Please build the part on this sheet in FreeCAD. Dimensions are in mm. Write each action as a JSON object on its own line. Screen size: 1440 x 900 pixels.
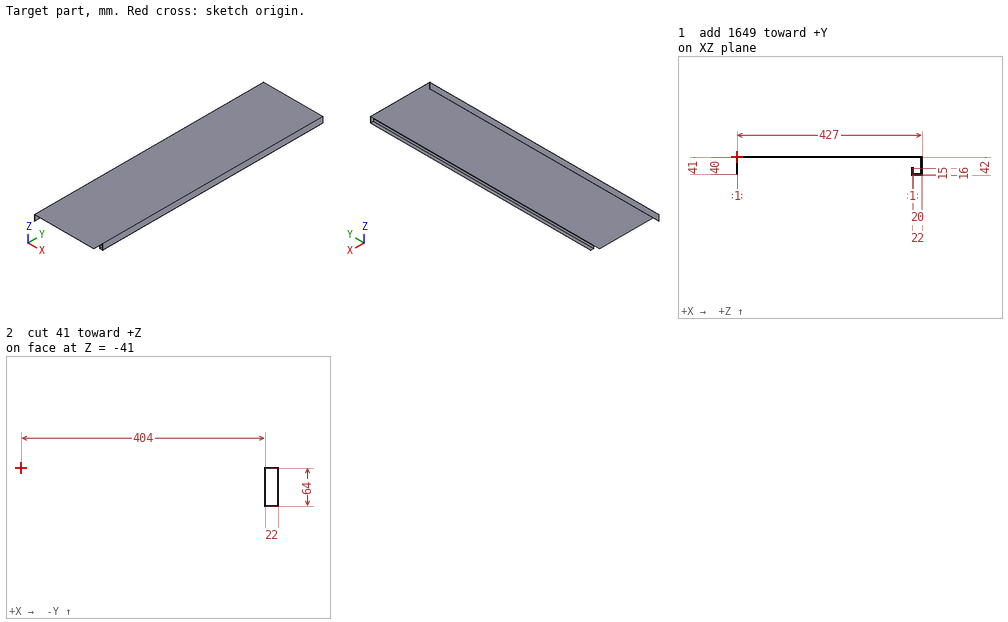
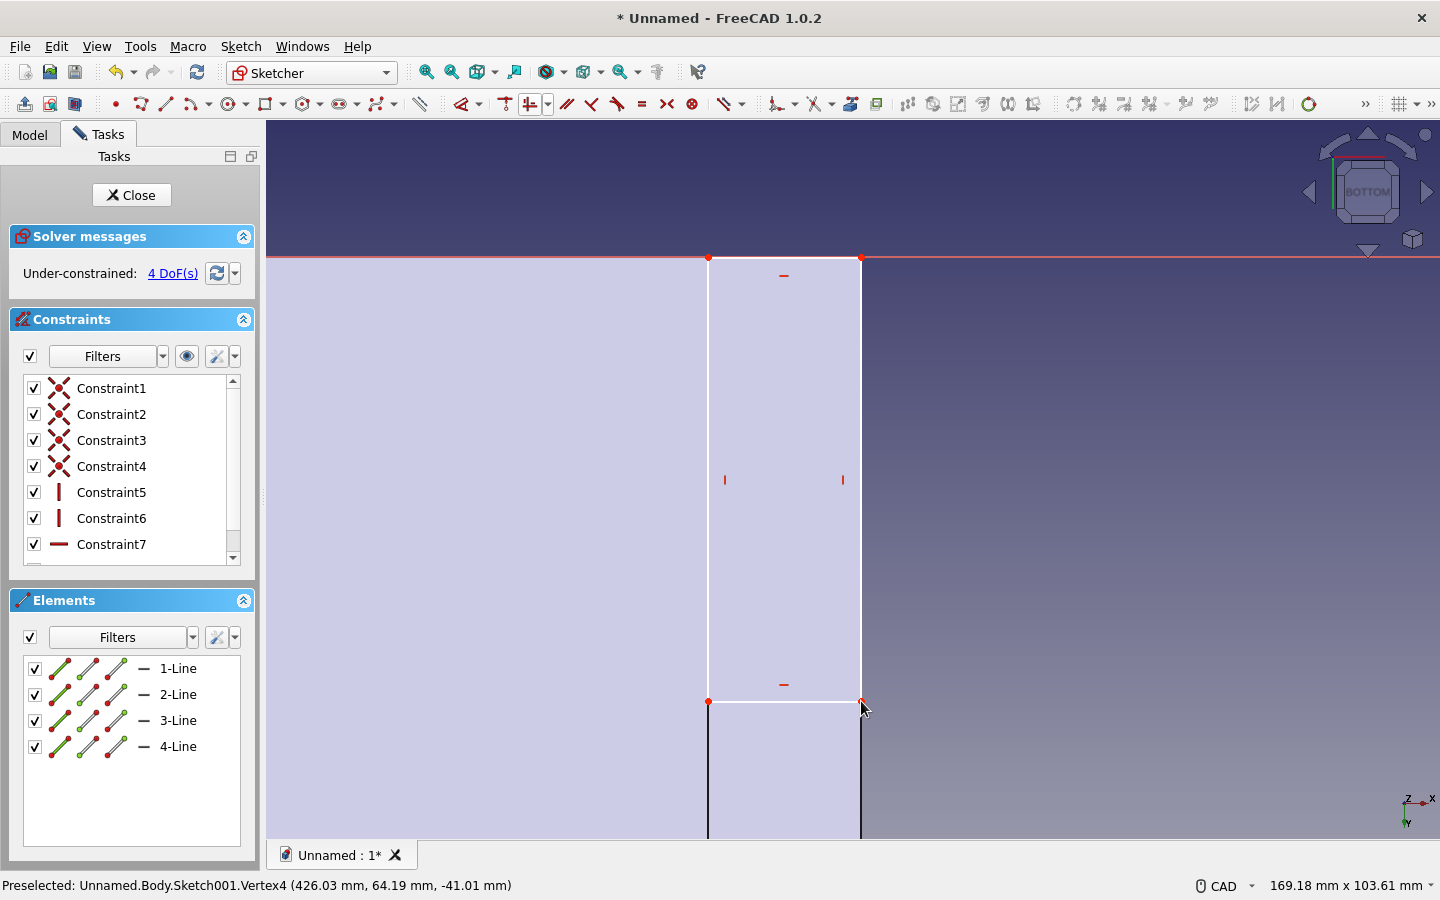
{"action": "left_click", "coordinate": [708, 258]}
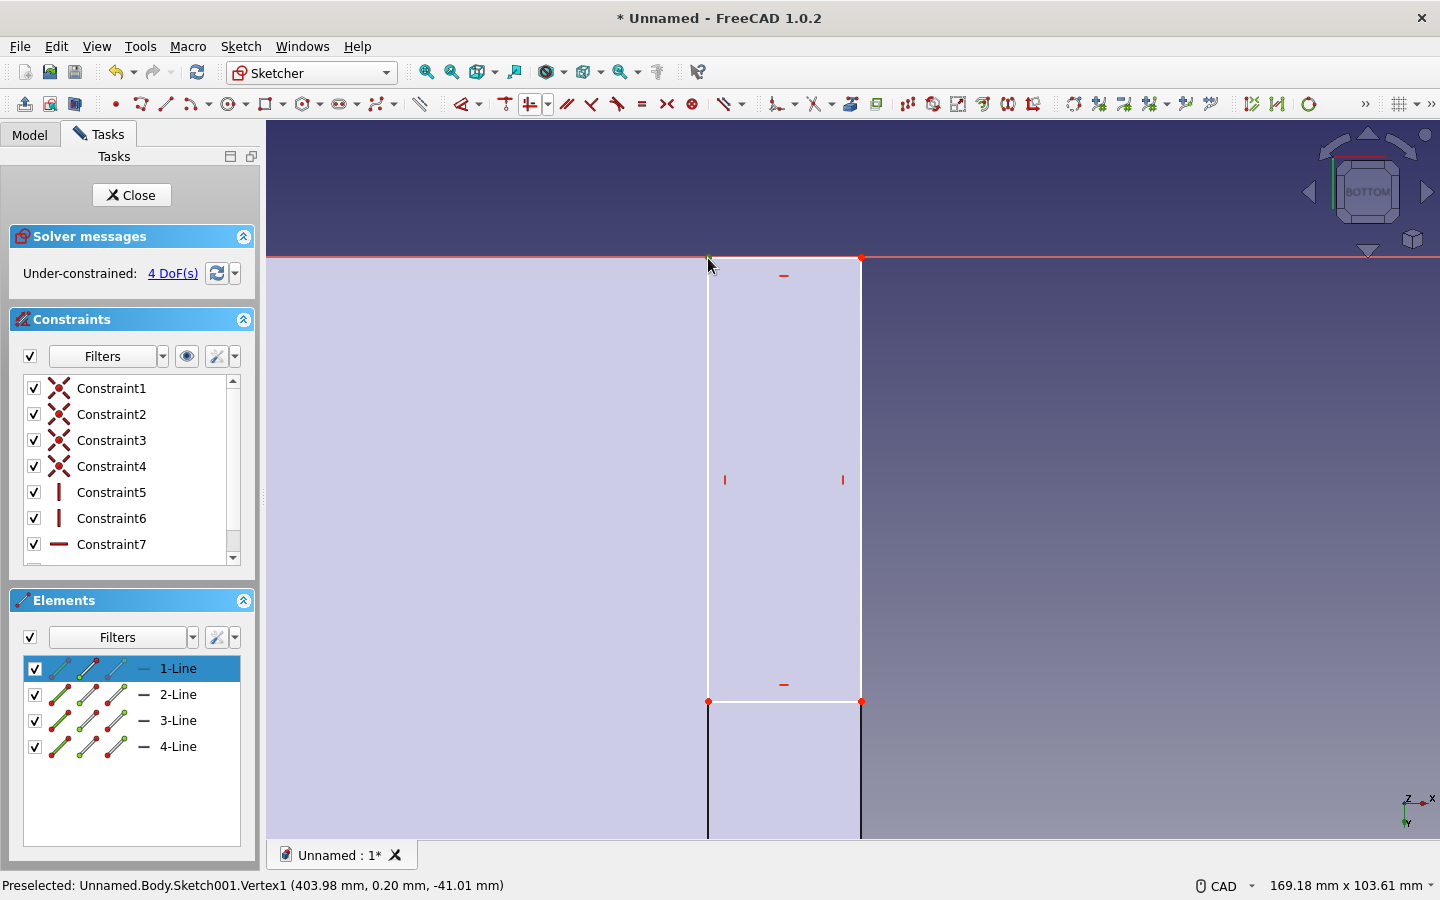
{"action": "left_click", "coordinate": [364, 257]}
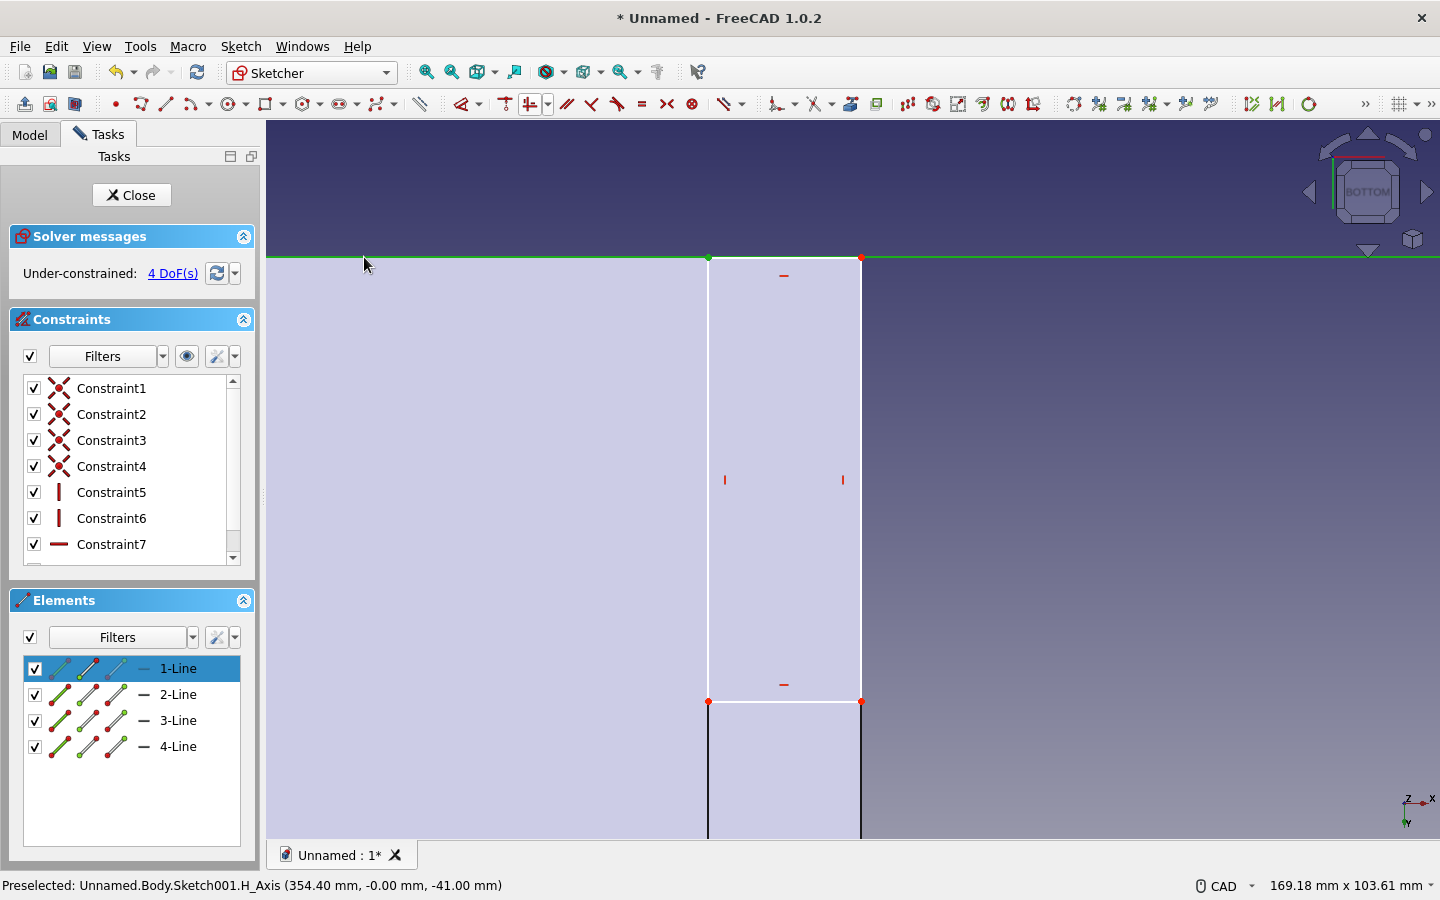
{"action": "left_click", "coordinate": [505, 104]}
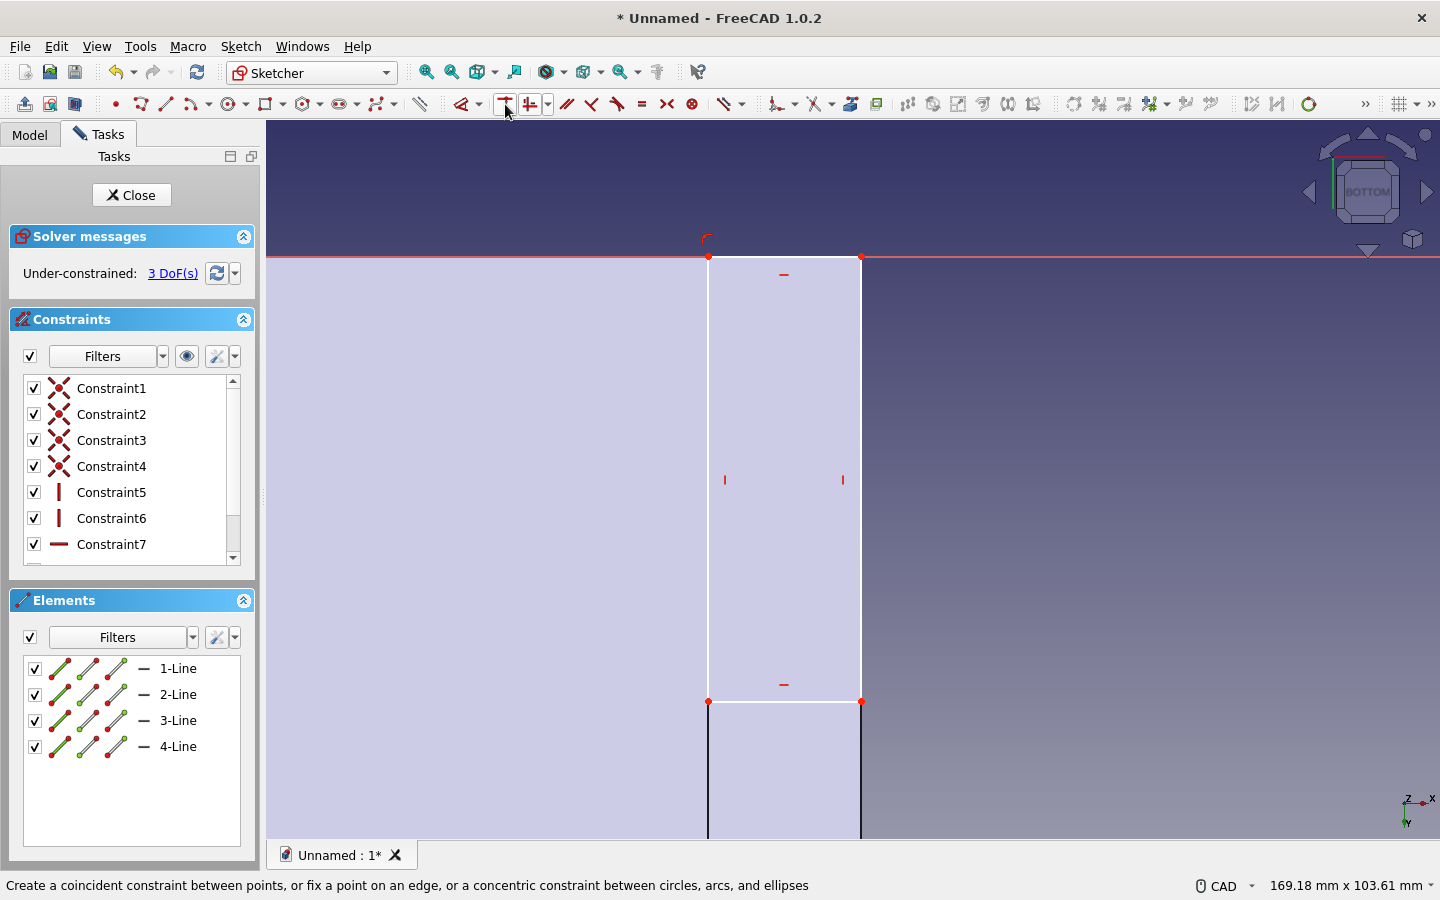
{"action": "left_click", "coordinate": [460, 104]}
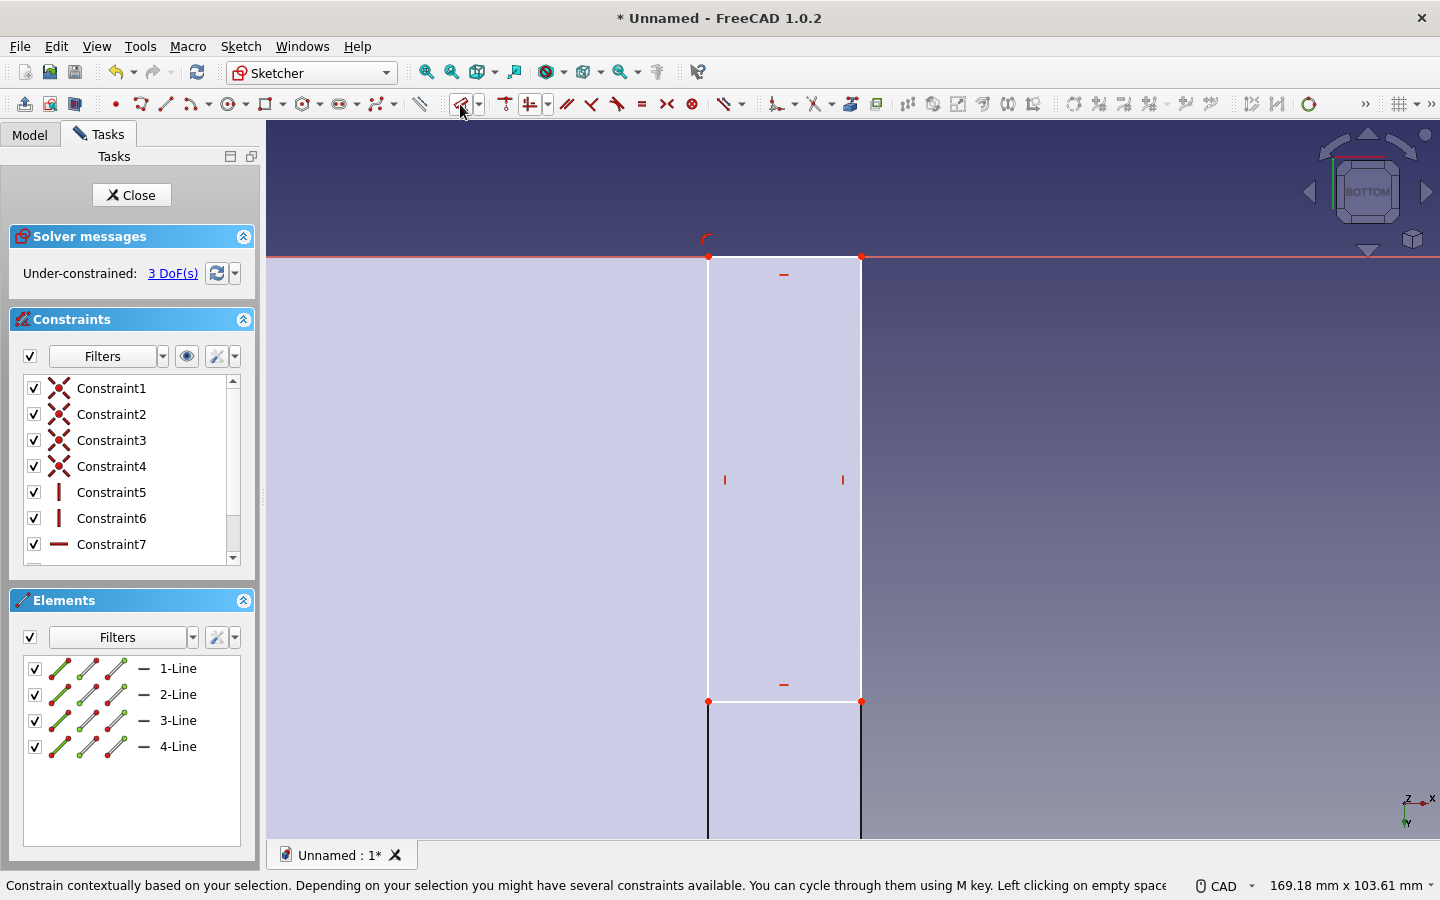
{"action": "left_click", "coordinate": [708, 390]}
{"action": "left_click", "coordinate": [674, 479]}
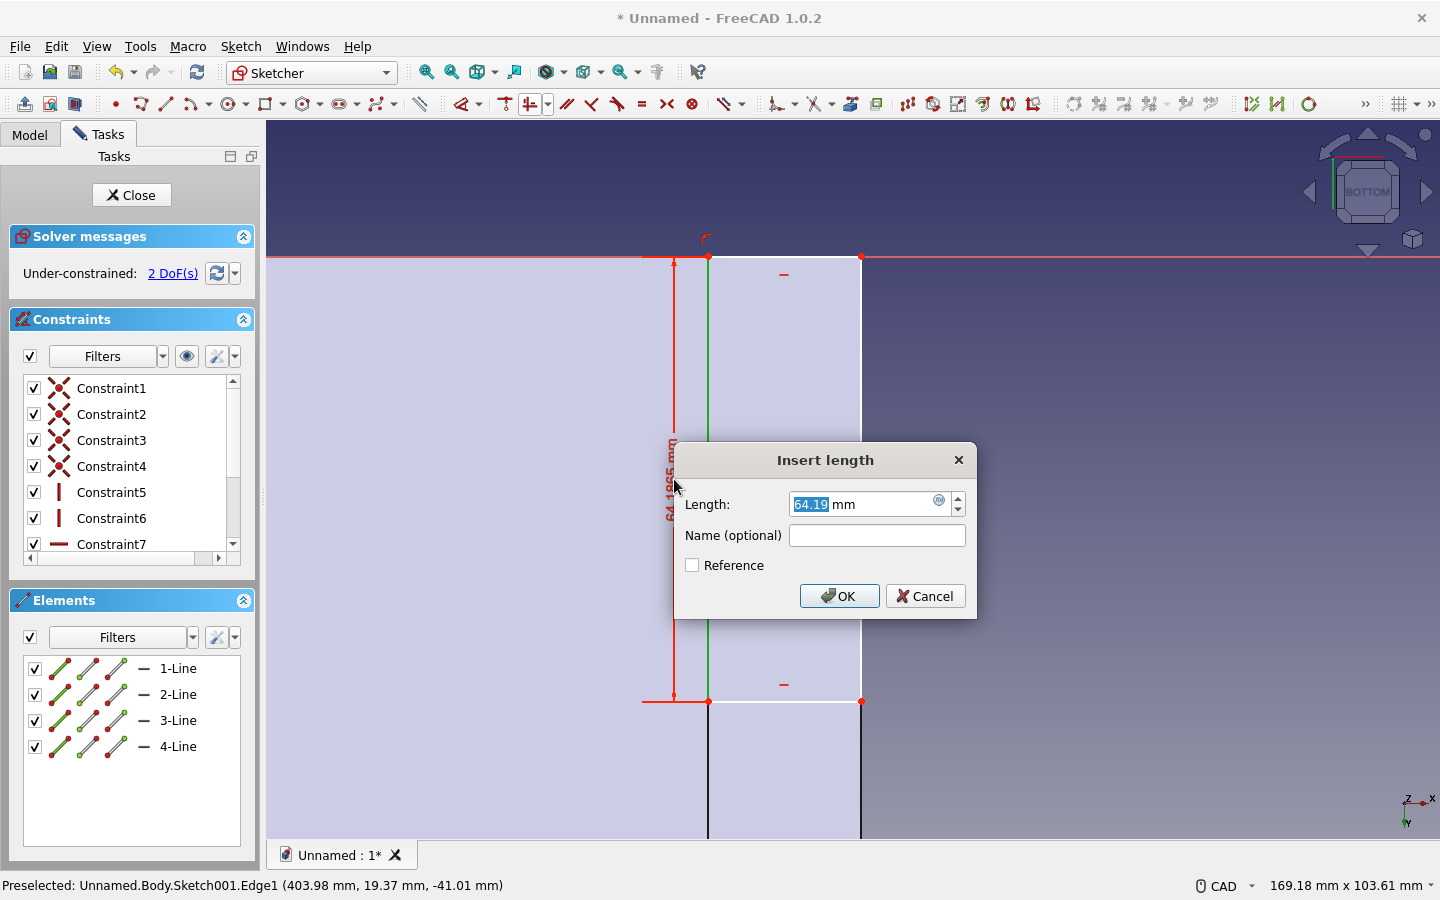
{"action": "type", "text": "64"}
{"action": "key", "text": "Return"}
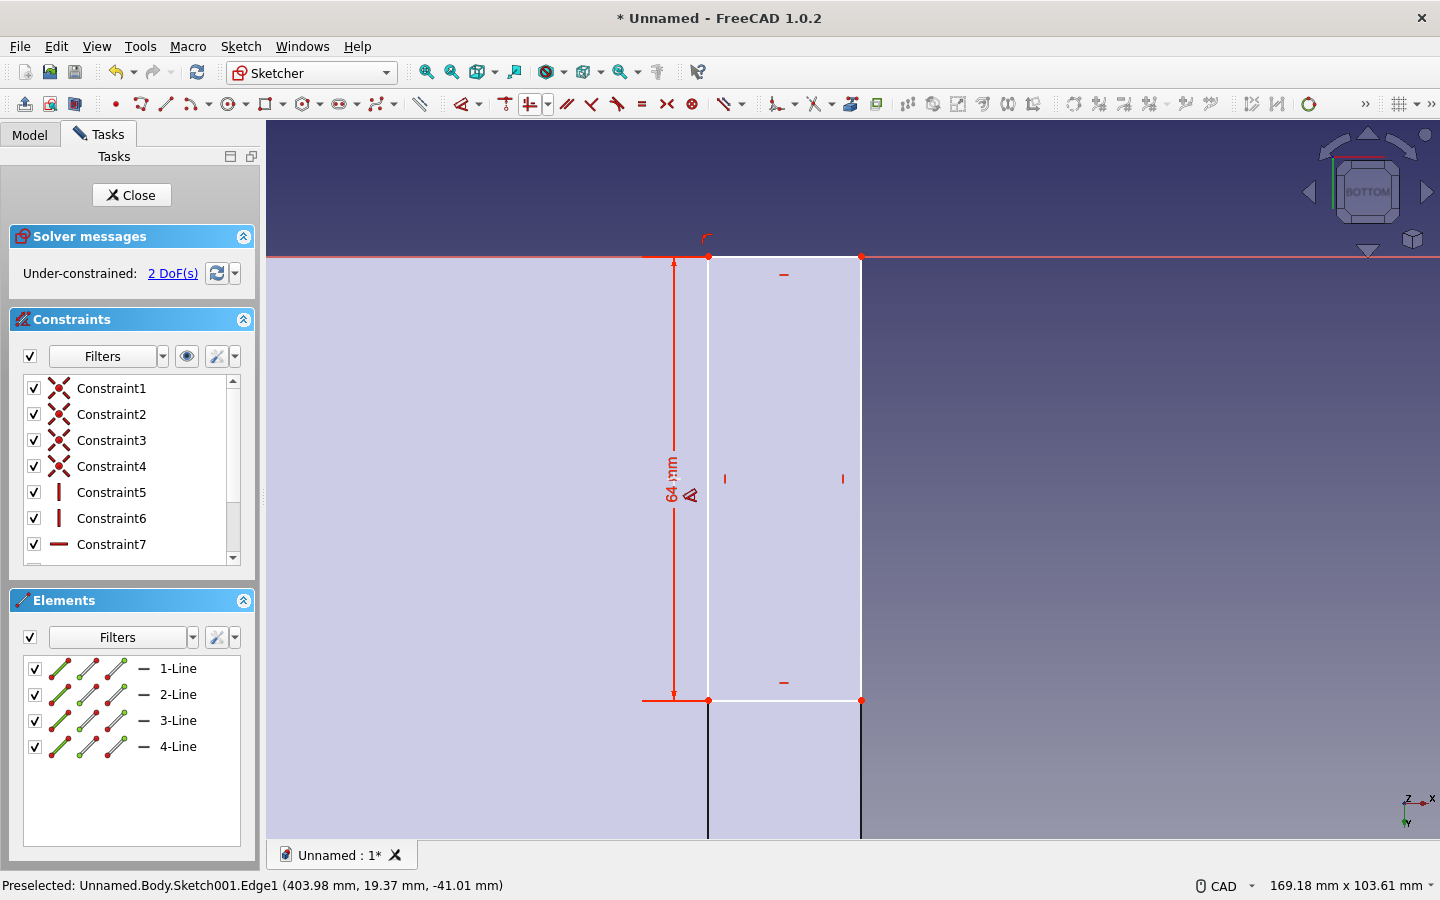
{"action": "left_click", "coordinate": [754, 701]}
{"action": "left_click", "coordinate": [784, 735]}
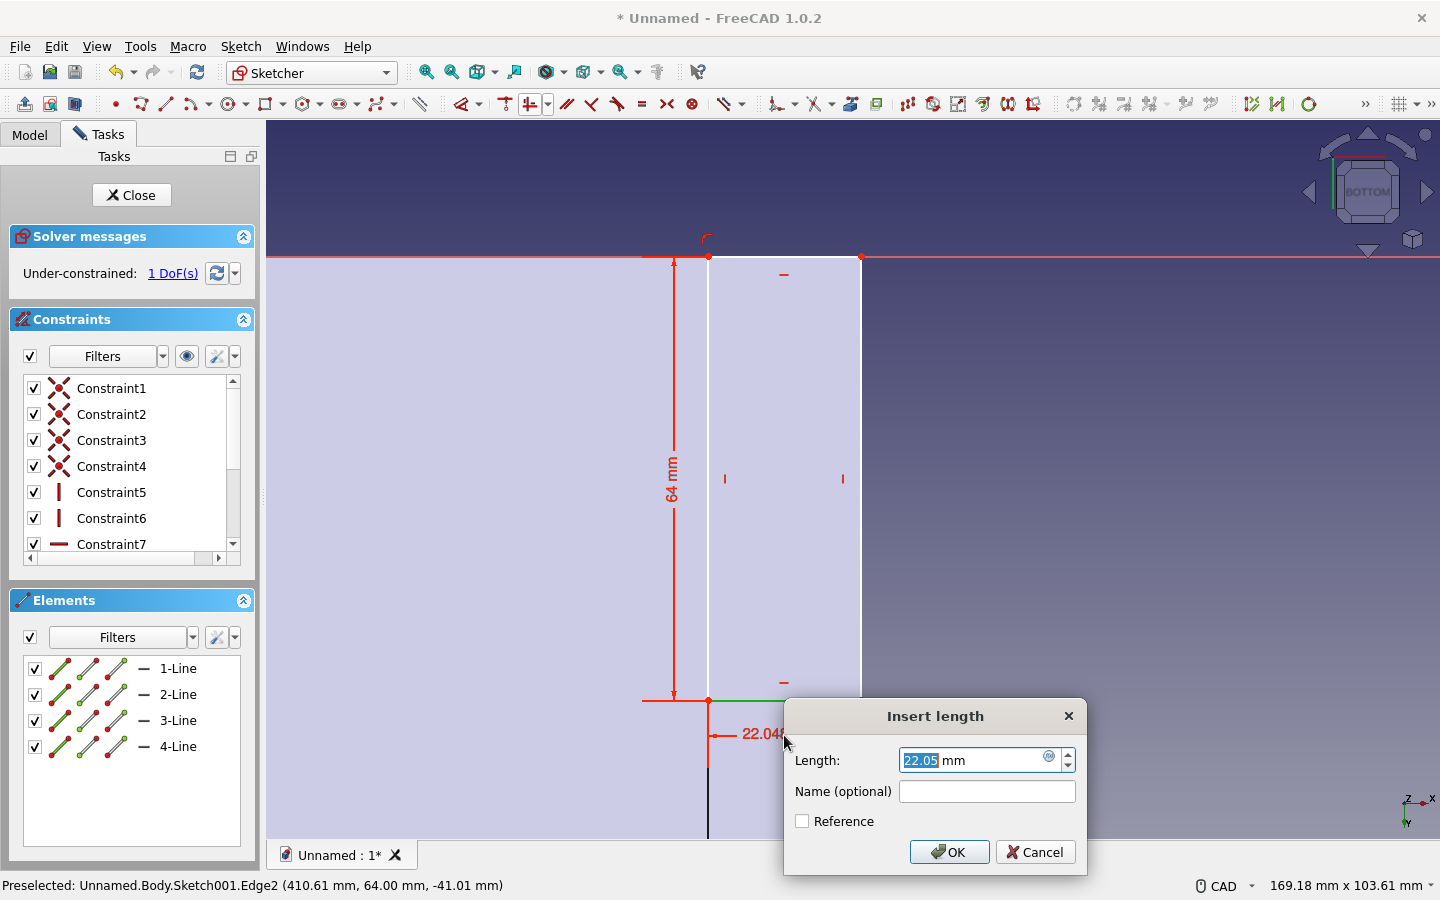
{"action": "type", "text": "22"}
{"action": "key", "text": "Return"}